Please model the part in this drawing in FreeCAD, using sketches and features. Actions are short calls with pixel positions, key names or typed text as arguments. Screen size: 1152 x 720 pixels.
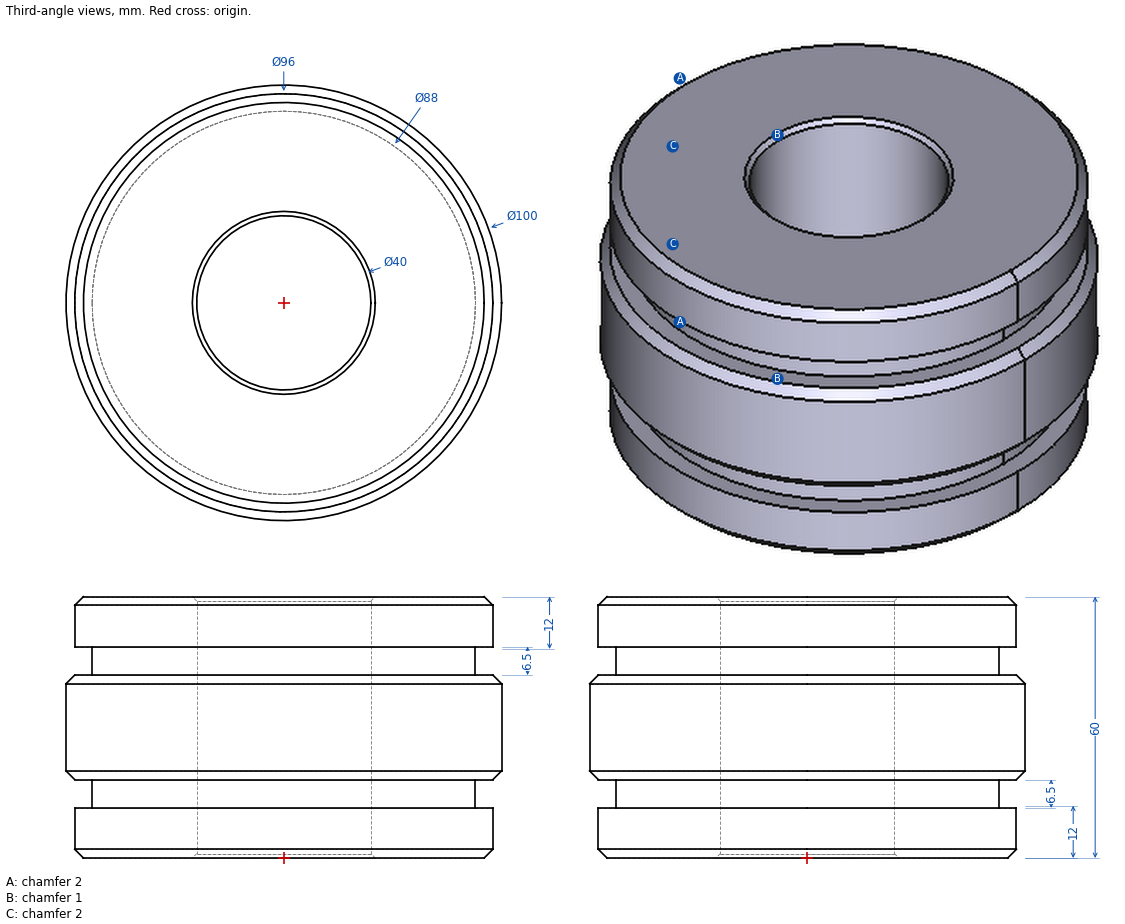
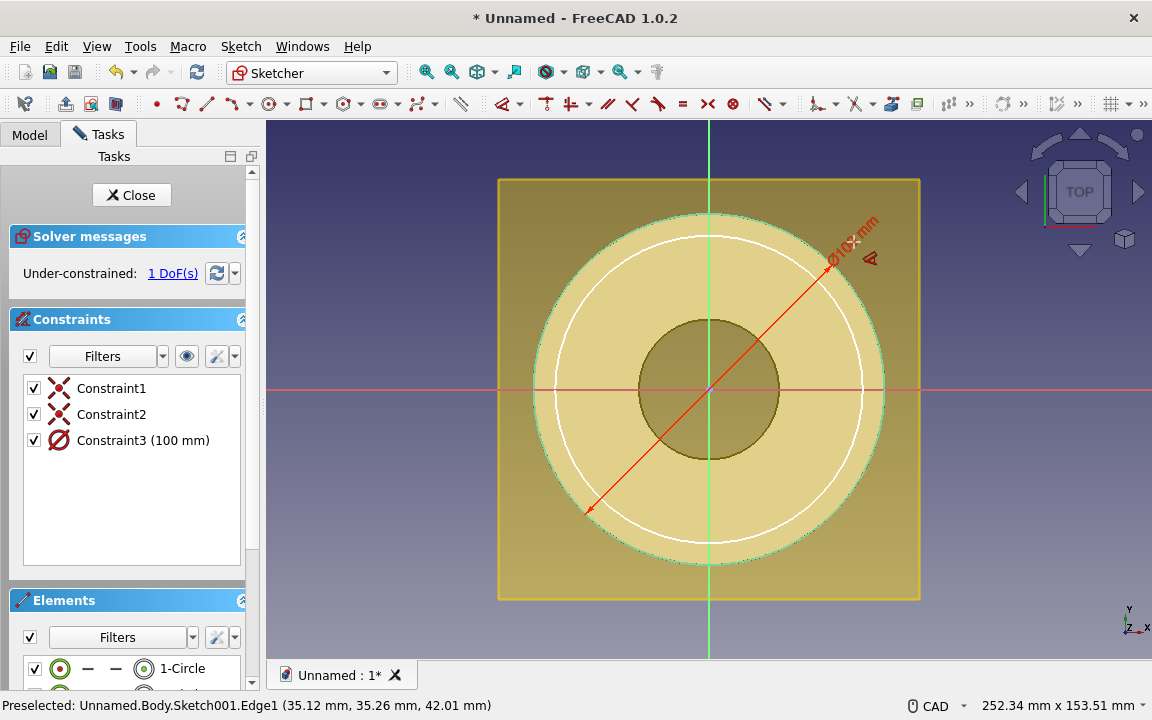
click(817, 280)
click(909, 329)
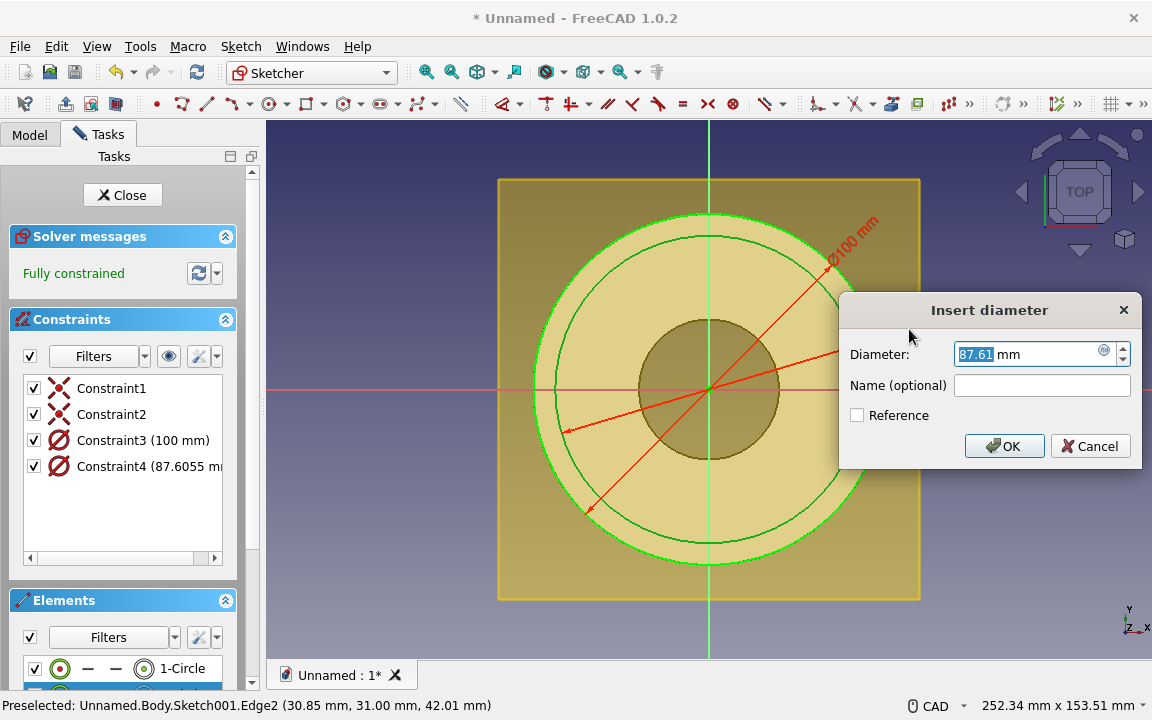
text(88)
key(Return)
key(Escape)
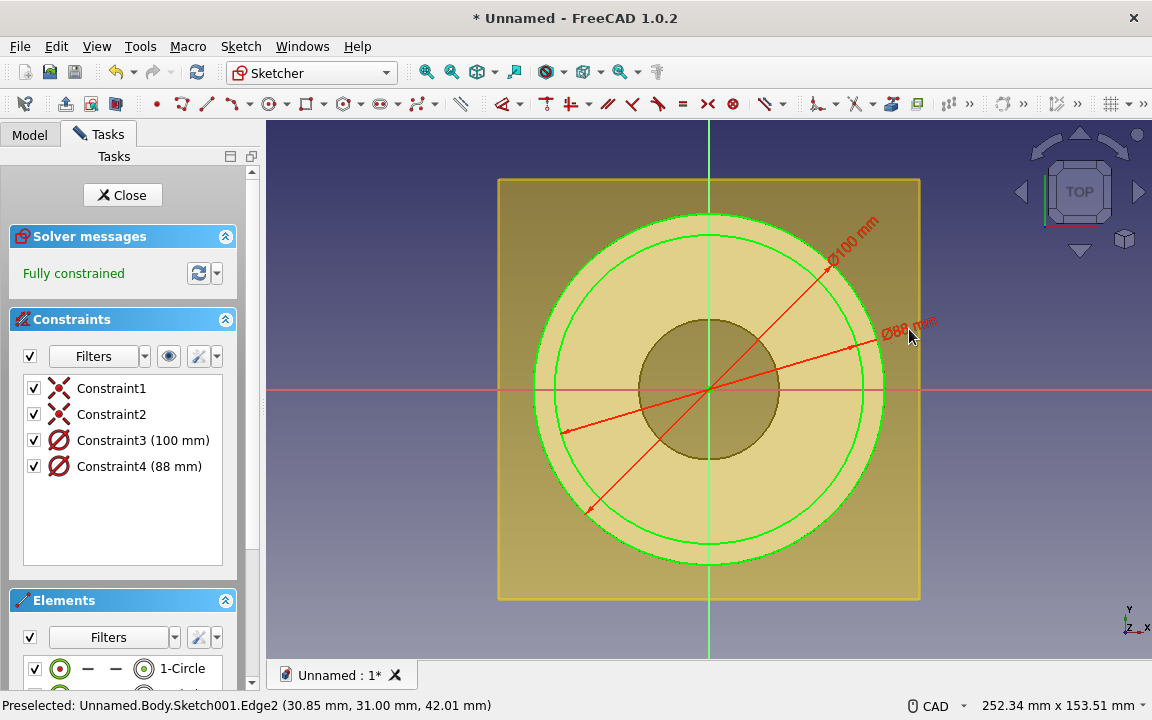
click(123, 195)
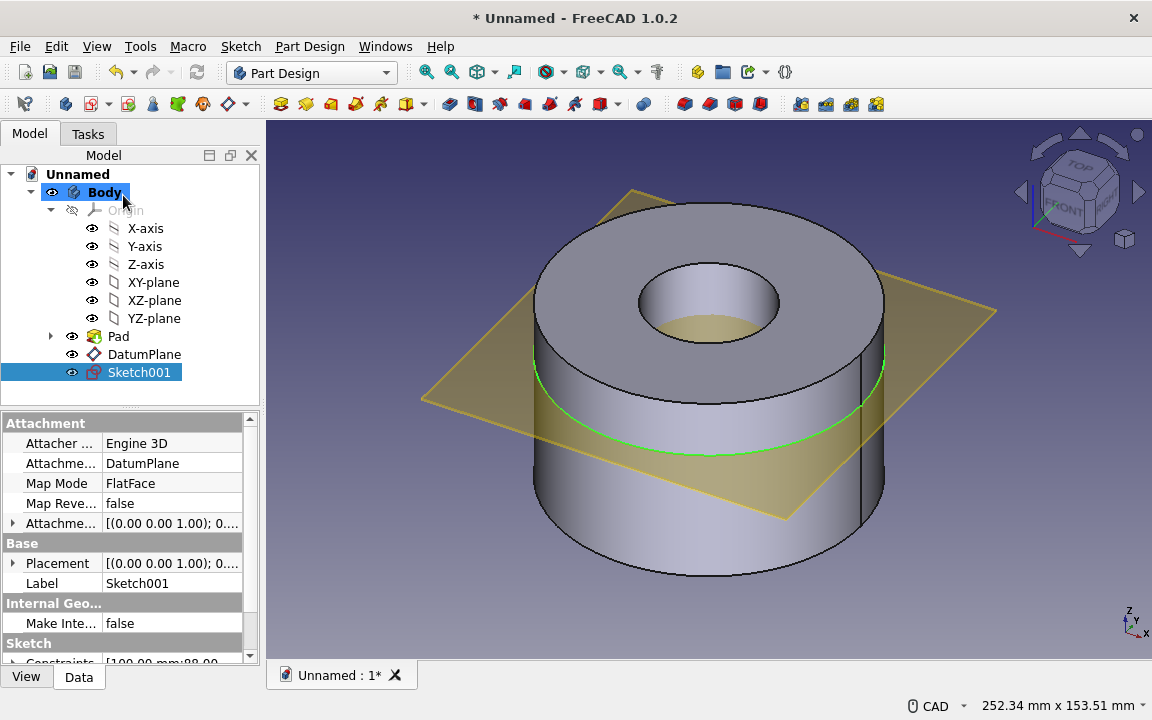
click(450, 104)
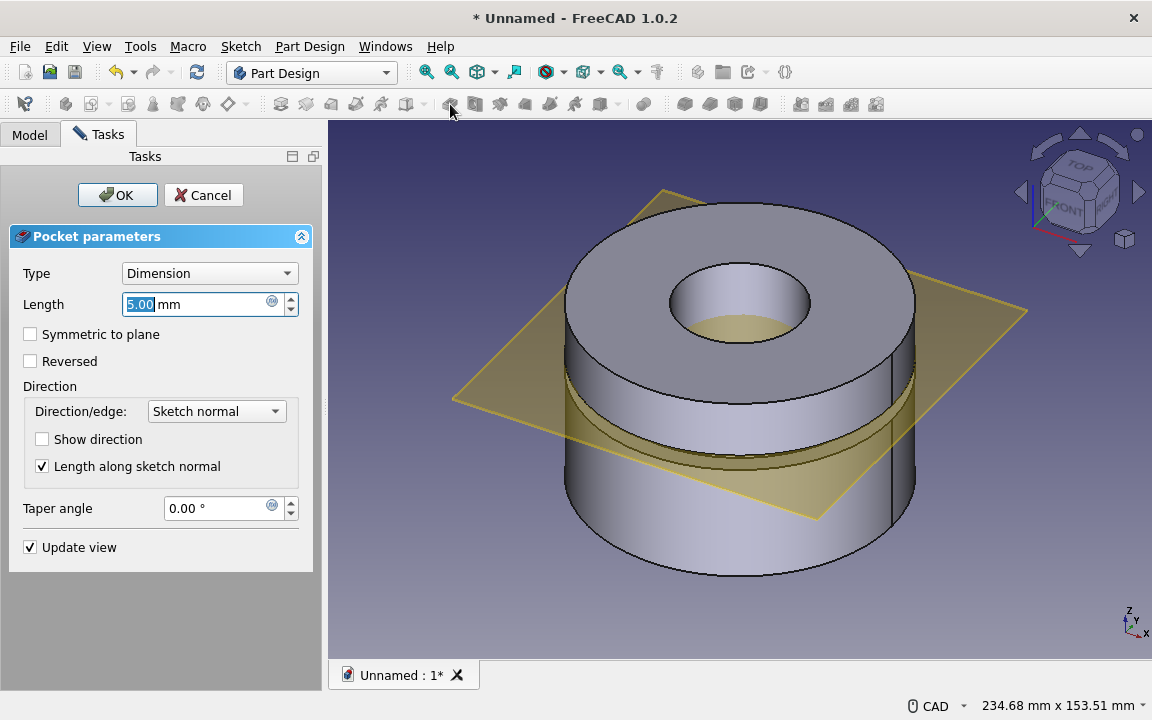
text(6.5)
key(Tab)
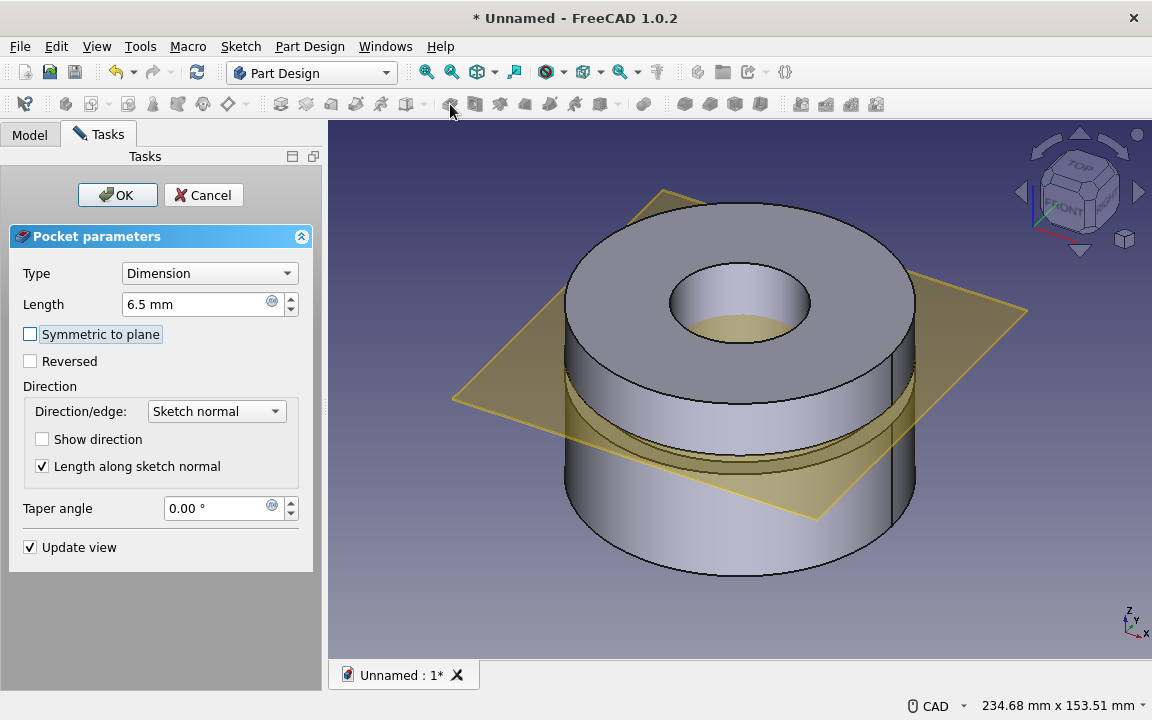
click(31, 361)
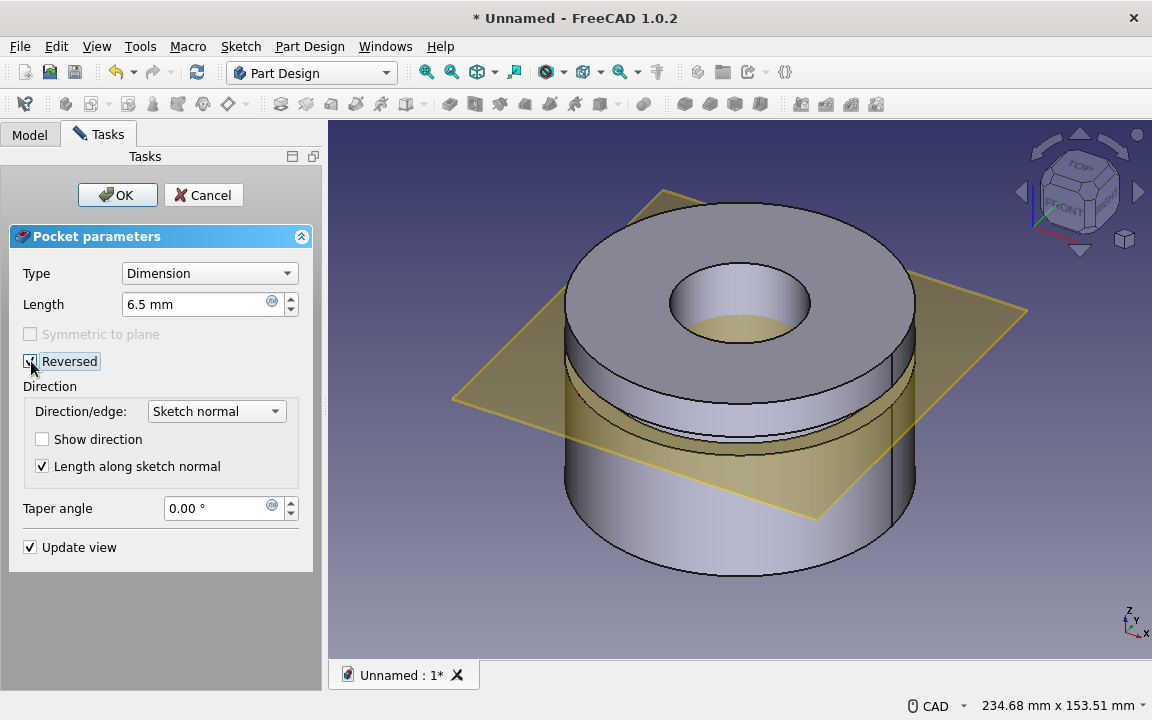
click(118, 195)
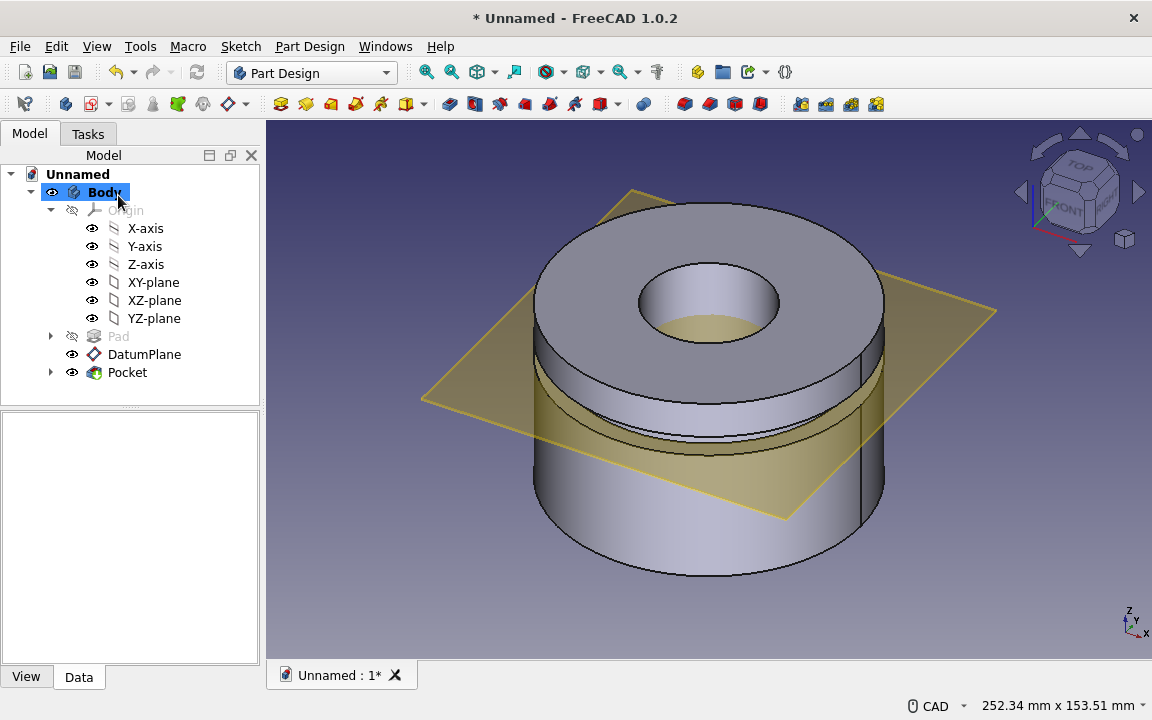
click(117, 354)
key(space)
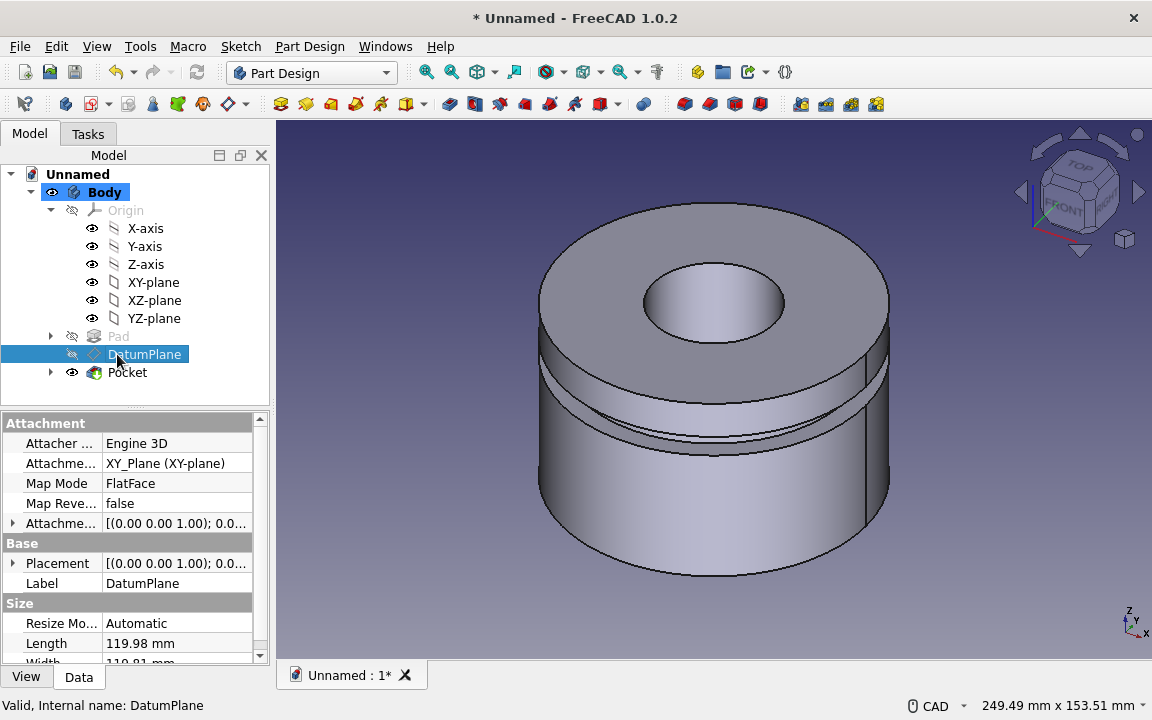
click(137, 282)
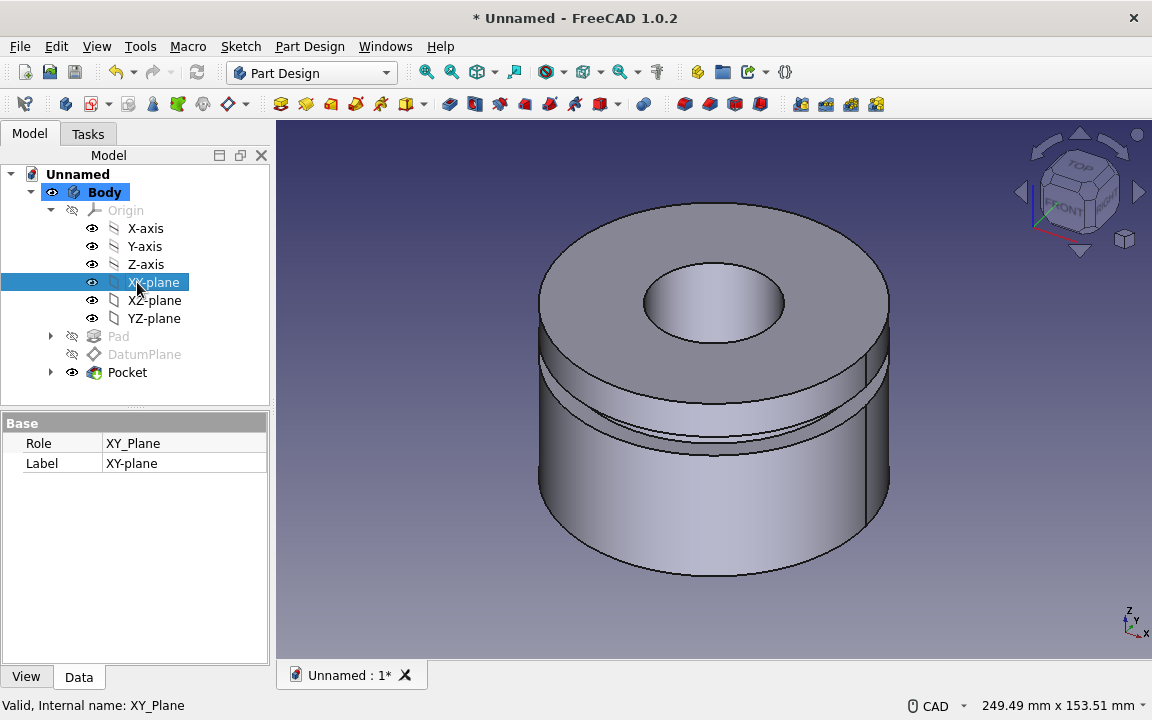
click(228, 104)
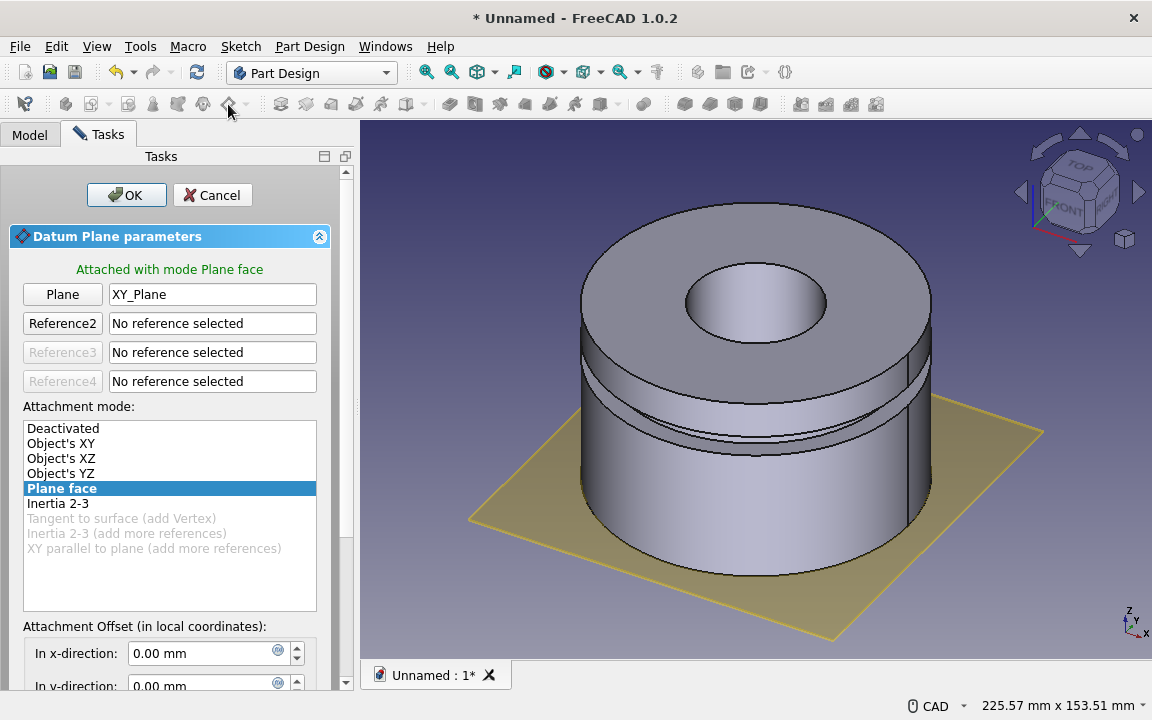
scroll(346, 428, down, 2)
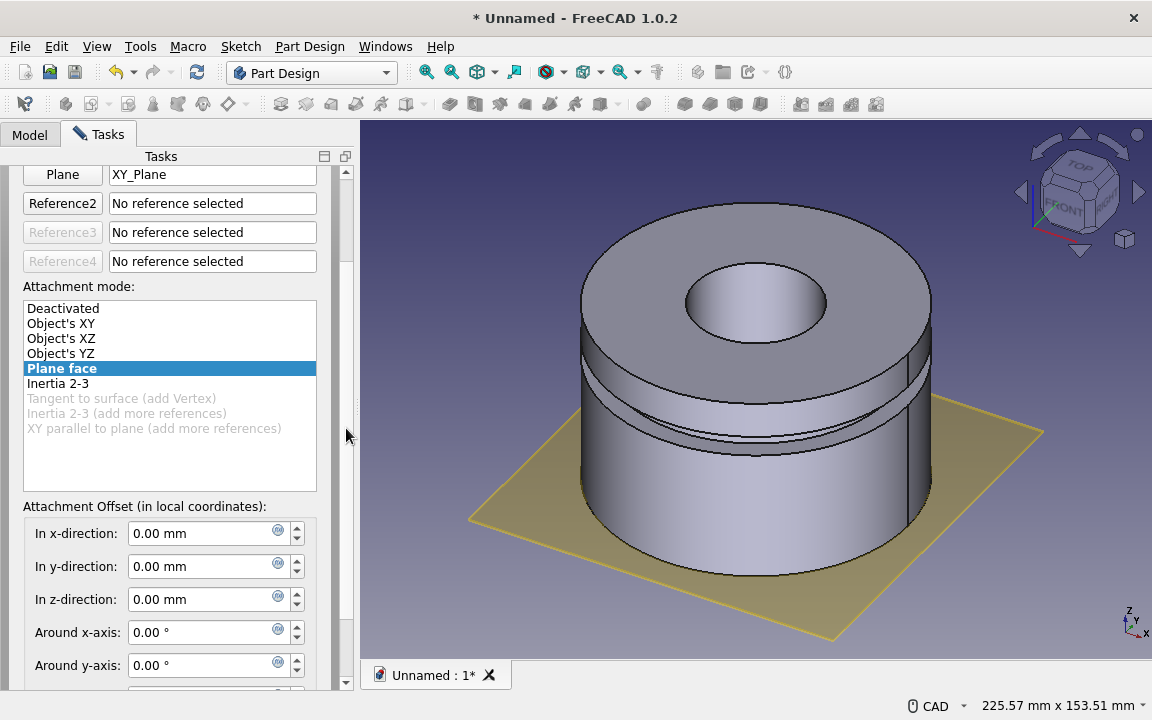
triple_click(210, 600)